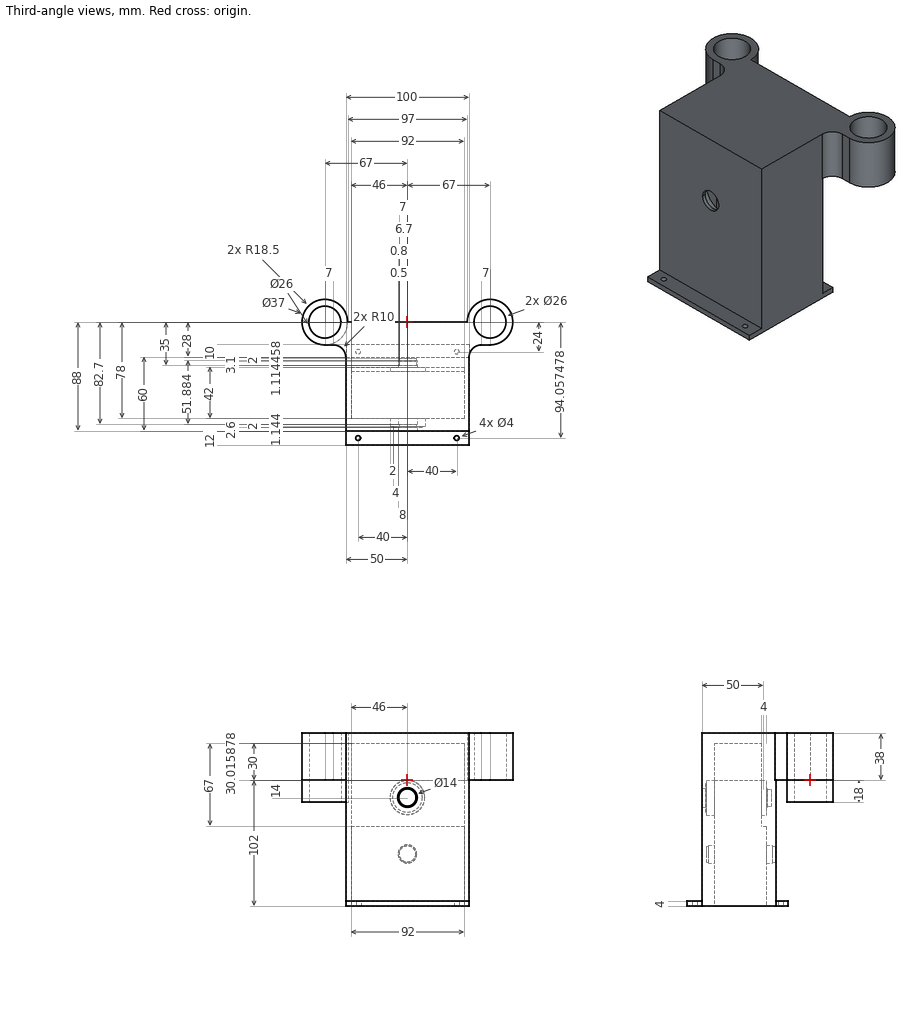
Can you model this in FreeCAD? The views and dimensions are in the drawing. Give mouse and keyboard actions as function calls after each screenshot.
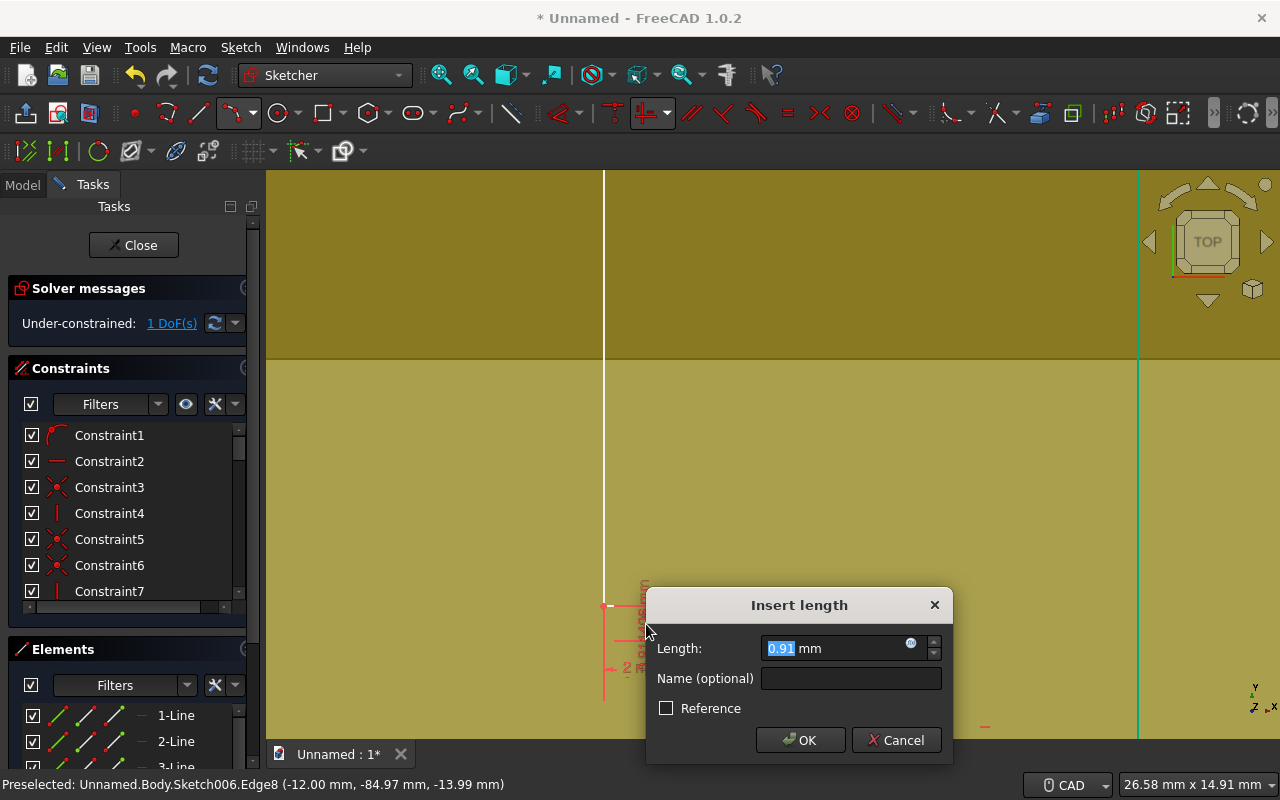
text(1.144)
key(Return)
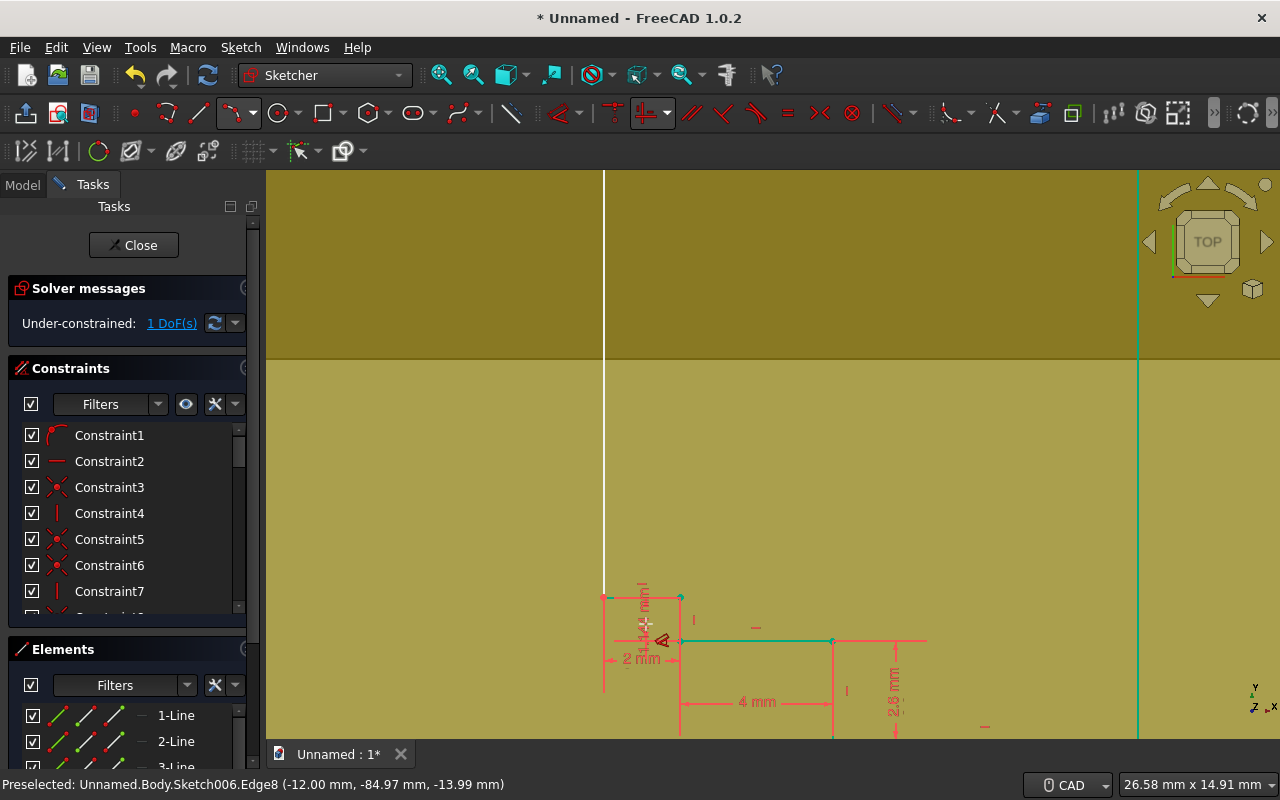
scroll(684, 628, down, 11)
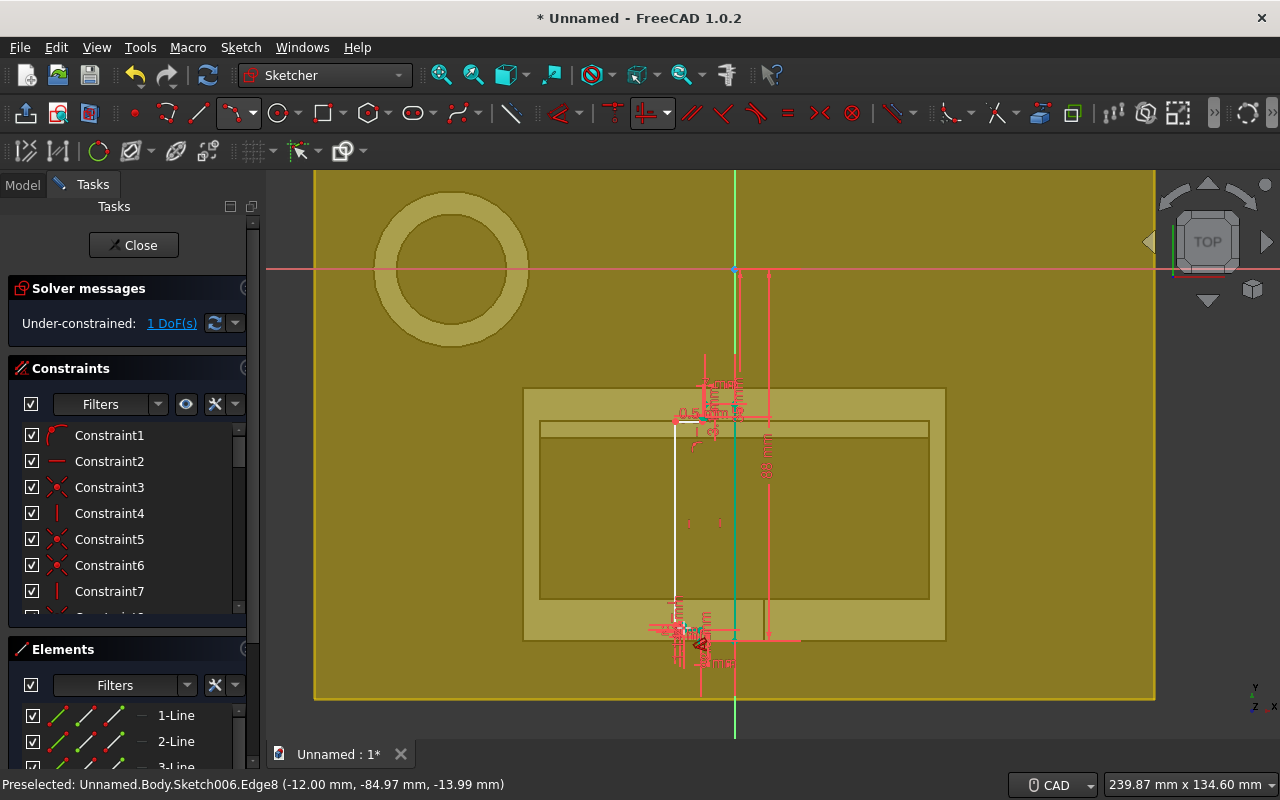
scroll(703, 419, up, 12)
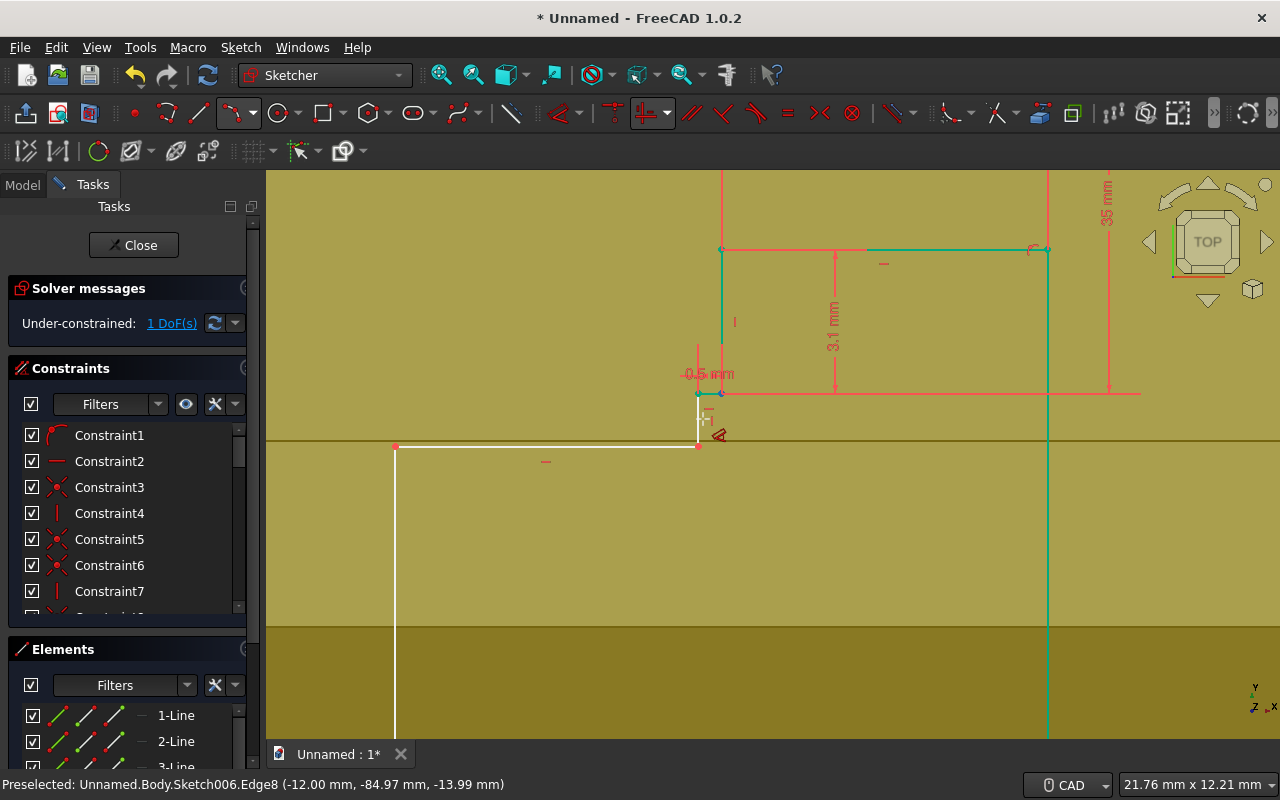
click(698, 410)
click(664, 420)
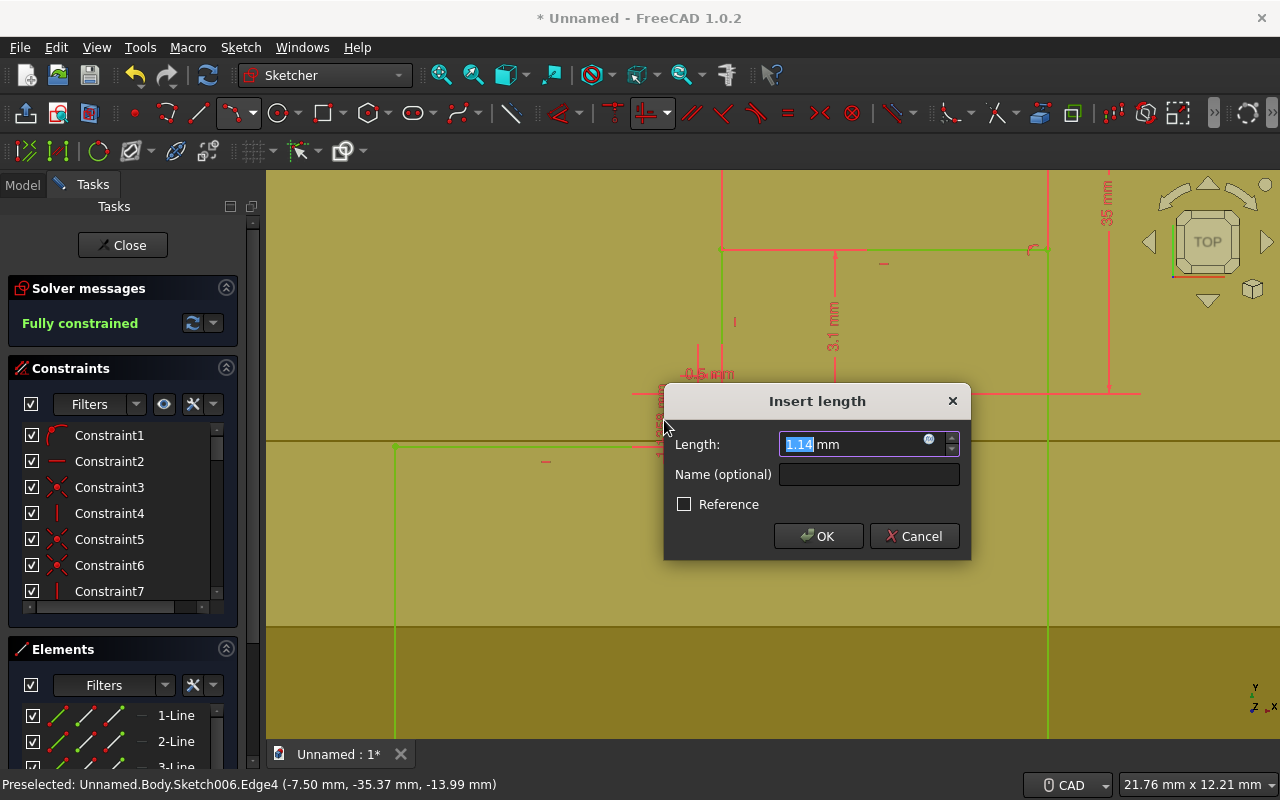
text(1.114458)
key(Return)
key(Escape)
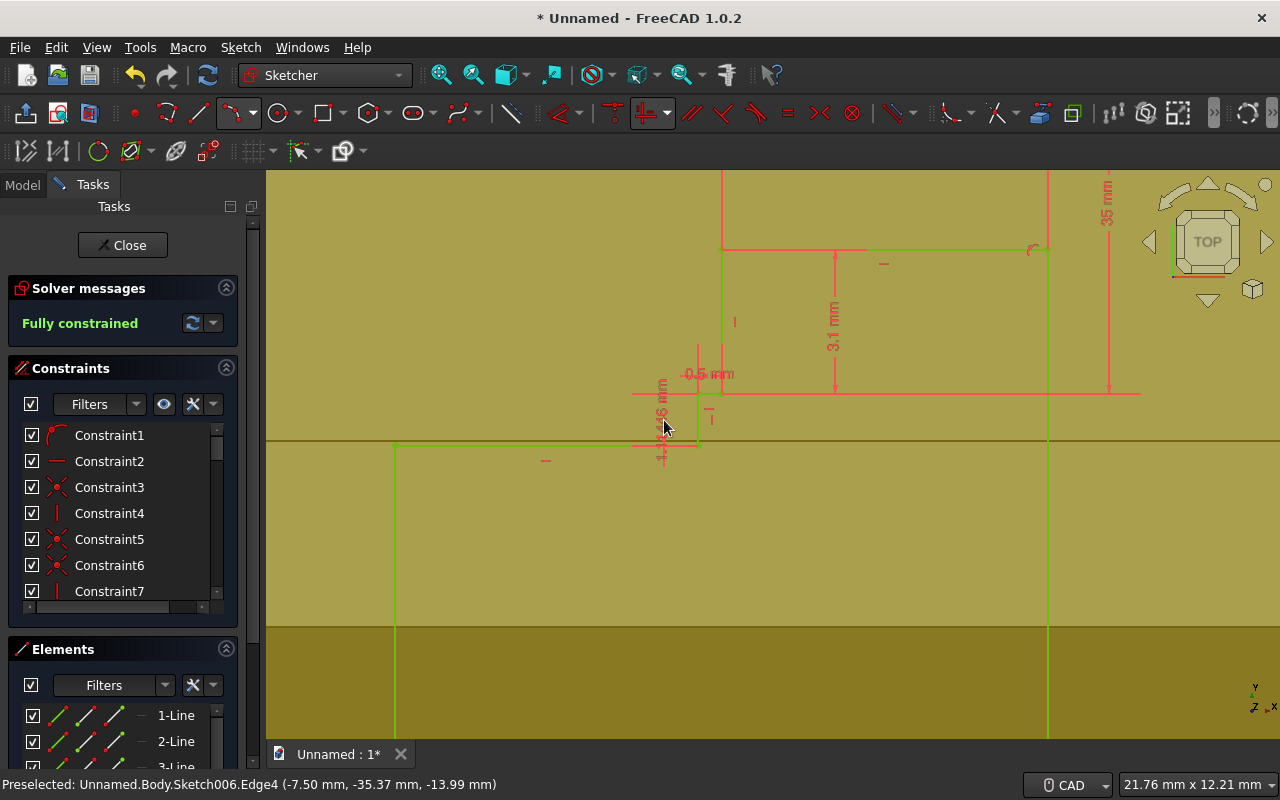
click(123, 245)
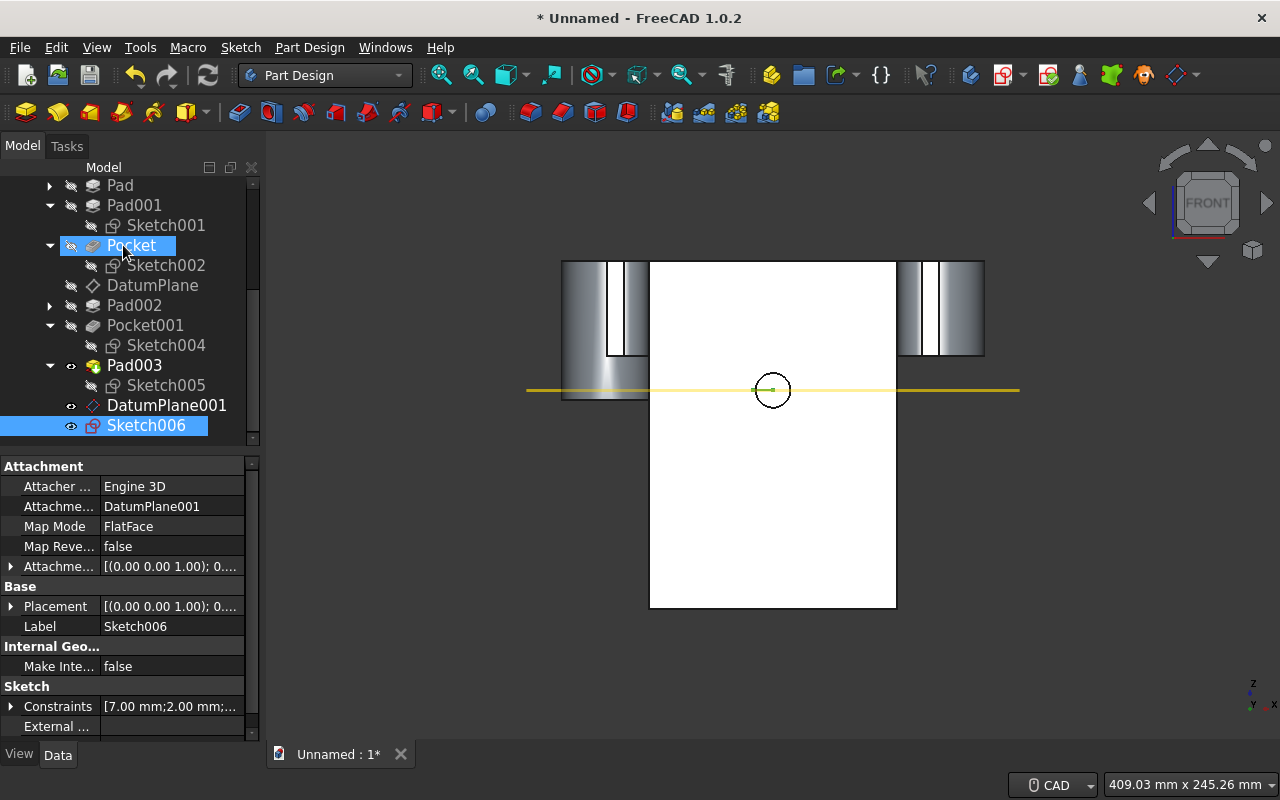
click(304, 112)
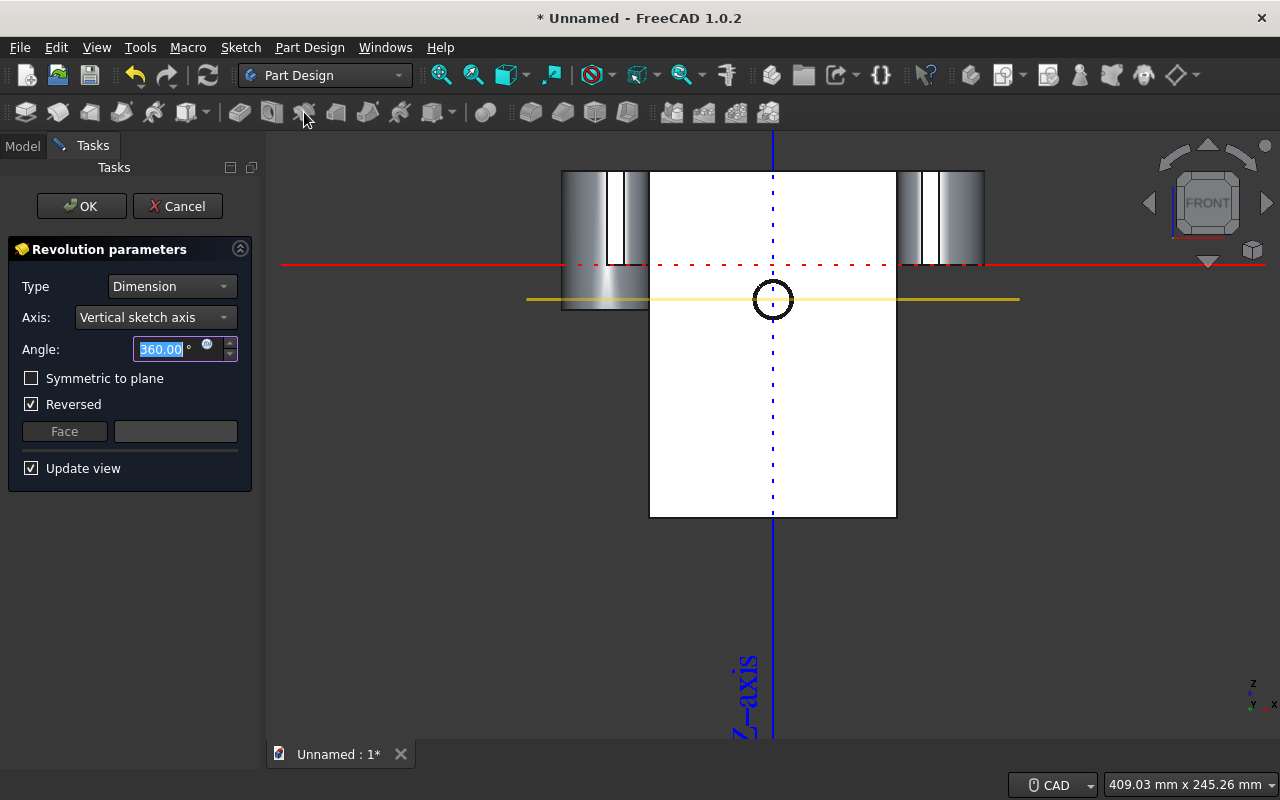
click(82, 206)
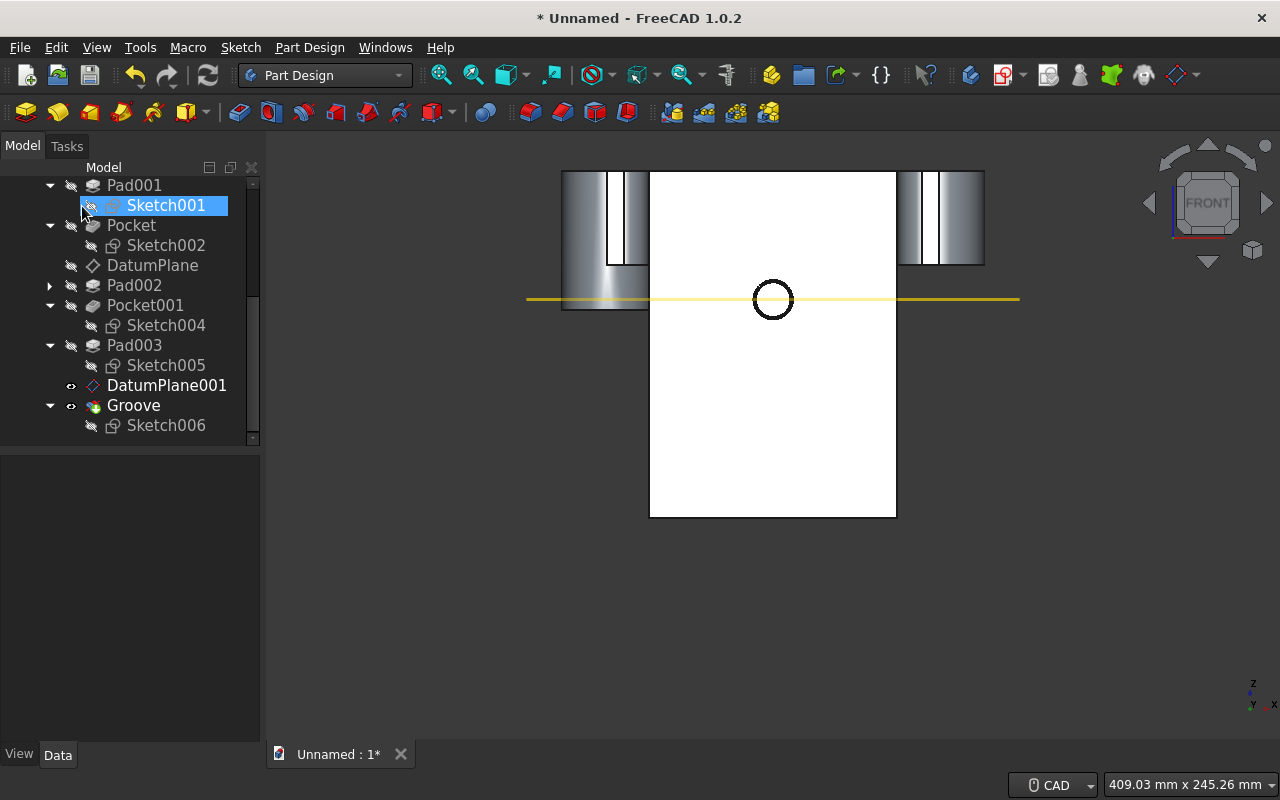
click(116, 386)
key(space)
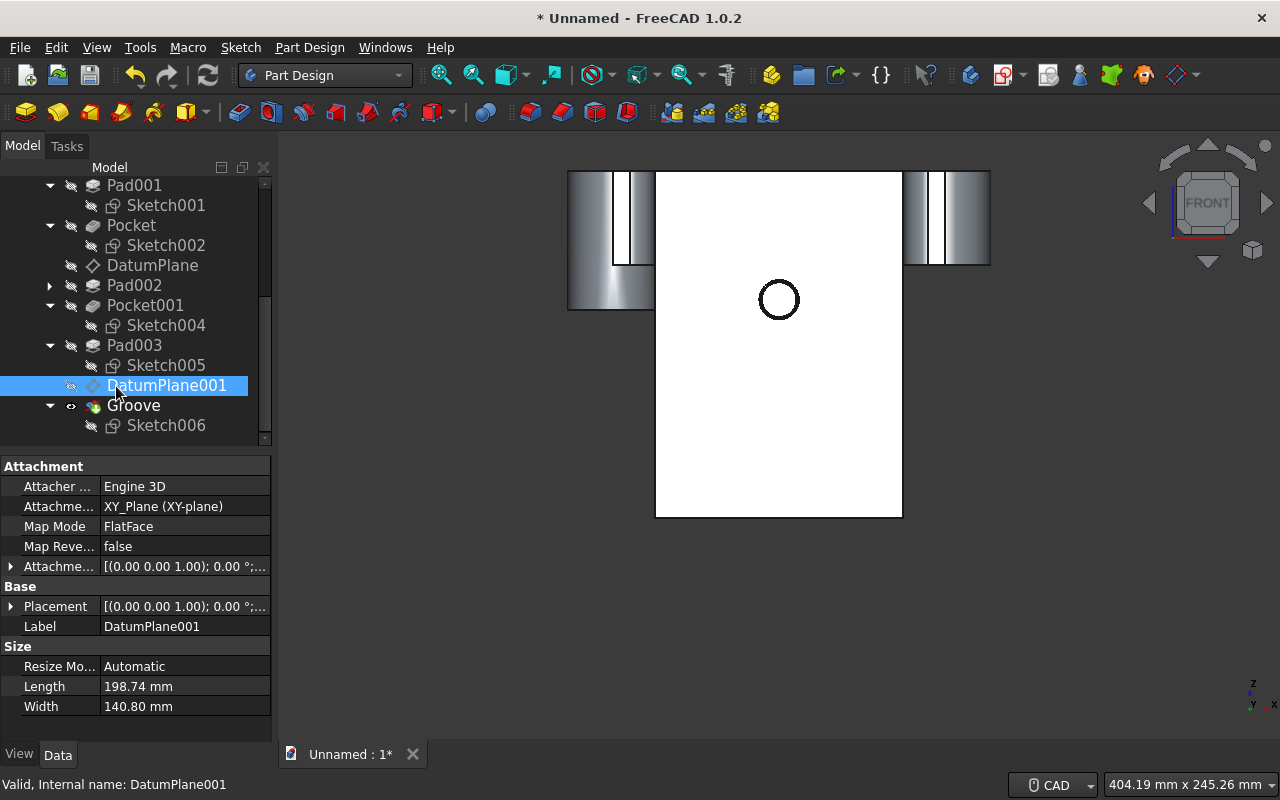
scroll(140, 301, down, 3)